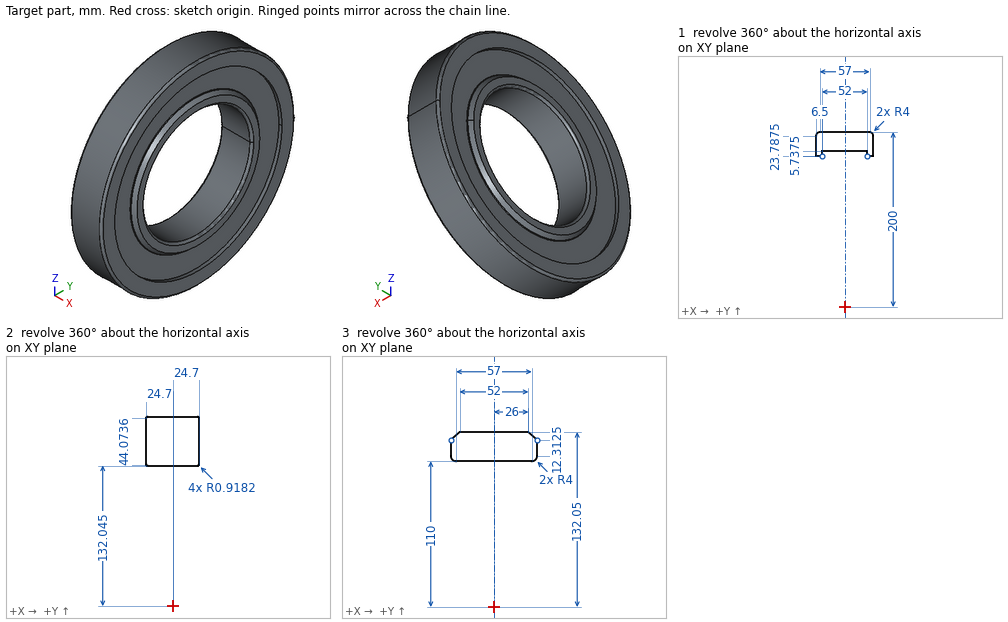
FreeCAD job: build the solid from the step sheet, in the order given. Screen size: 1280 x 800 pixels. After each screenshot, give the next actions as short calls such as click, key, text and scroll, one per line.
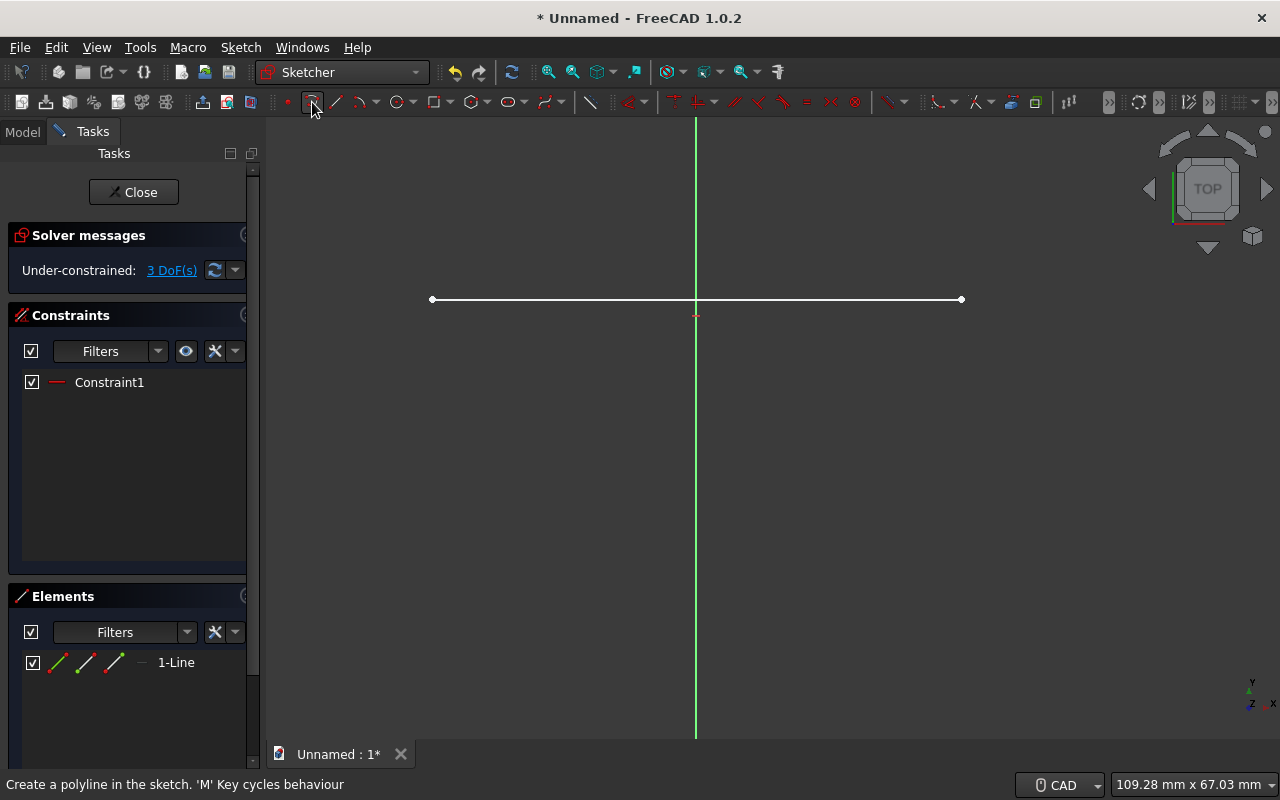
click(395, 336)
click(395, 557)
click(455, 557)
click(455, 503)
click(938, 503)
click(938, 557)
click(998, 557)
click(998, 336)
right_click(998, 336)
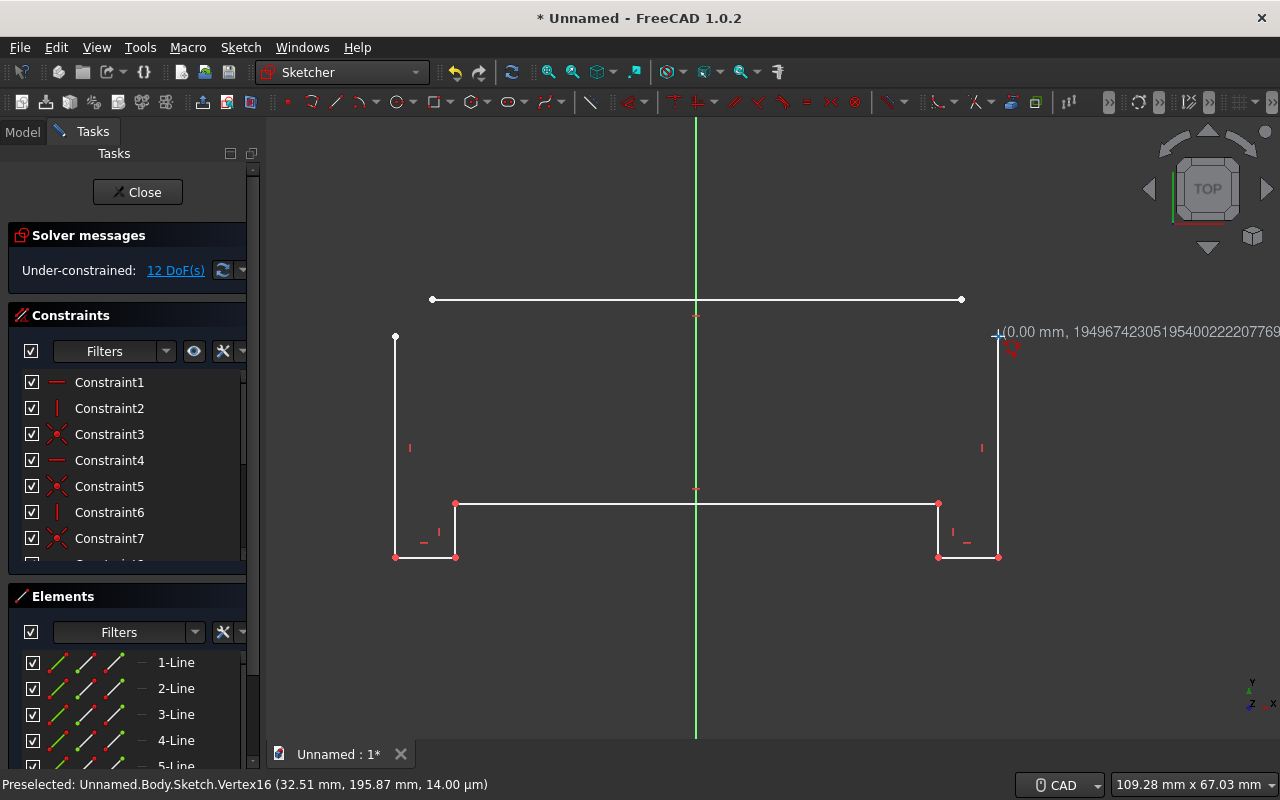
click(378, 102)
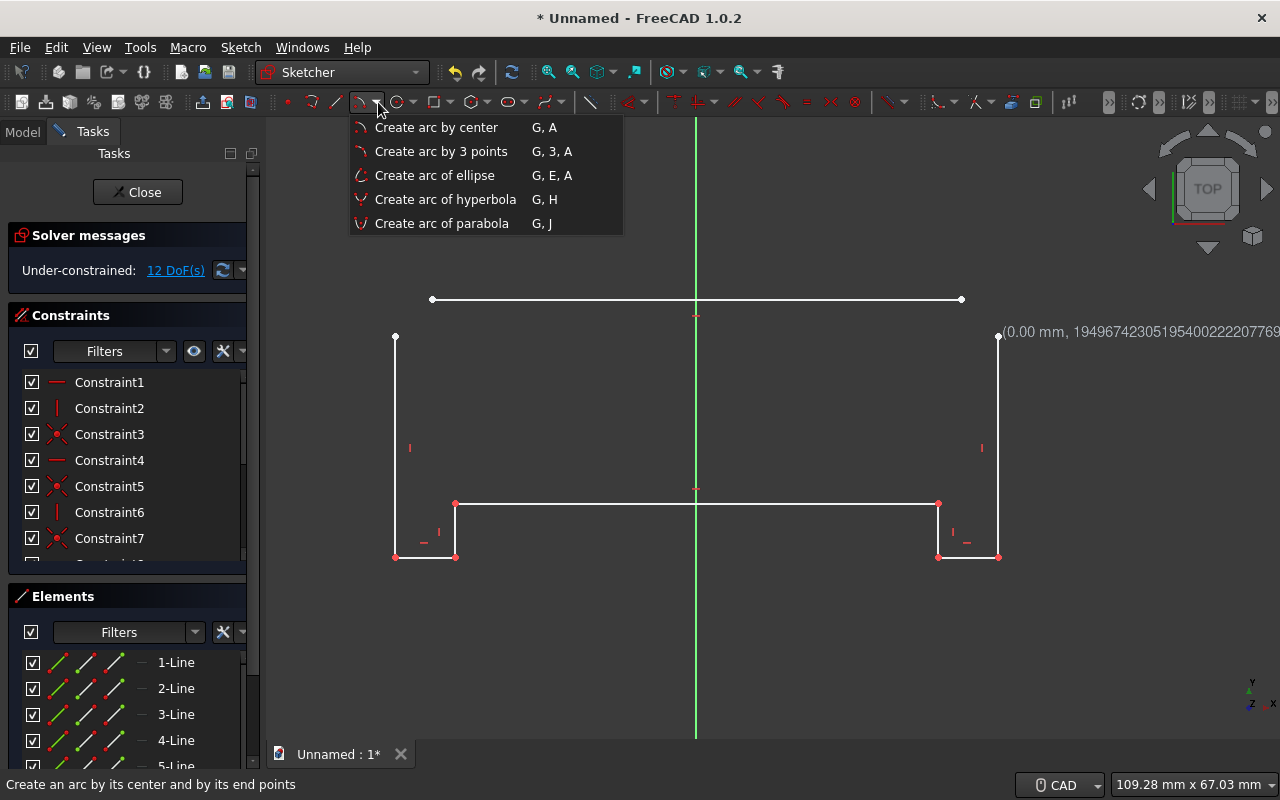
click(486, 151)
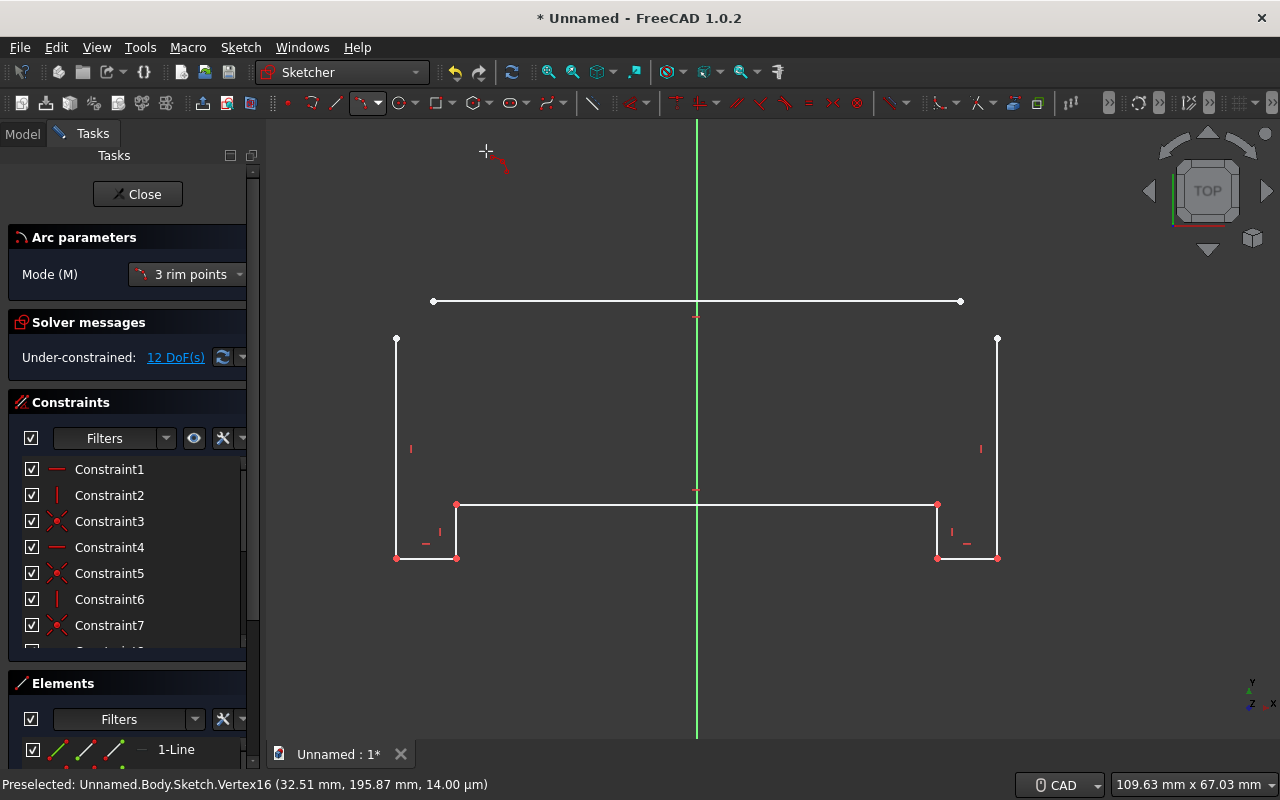
click(433, 301)
click(396, 338)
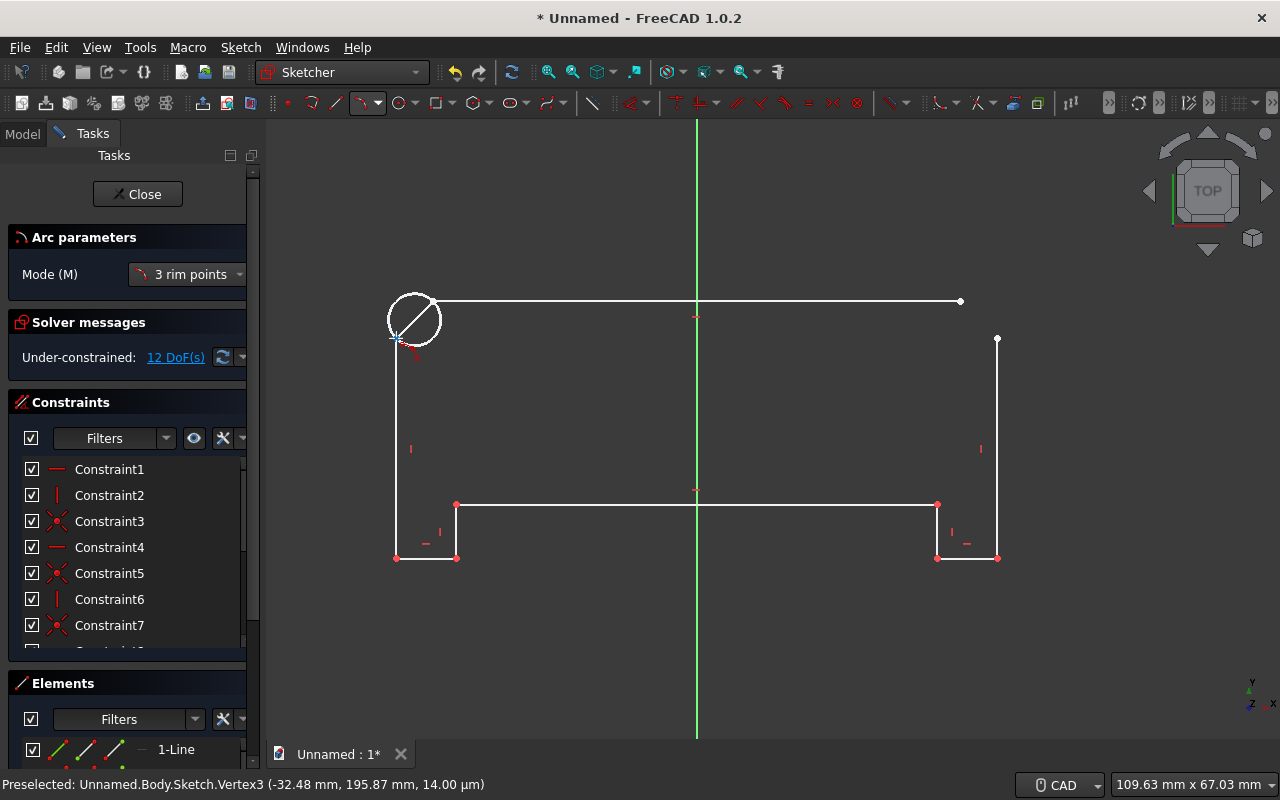
scroll(407, 311, up, 2)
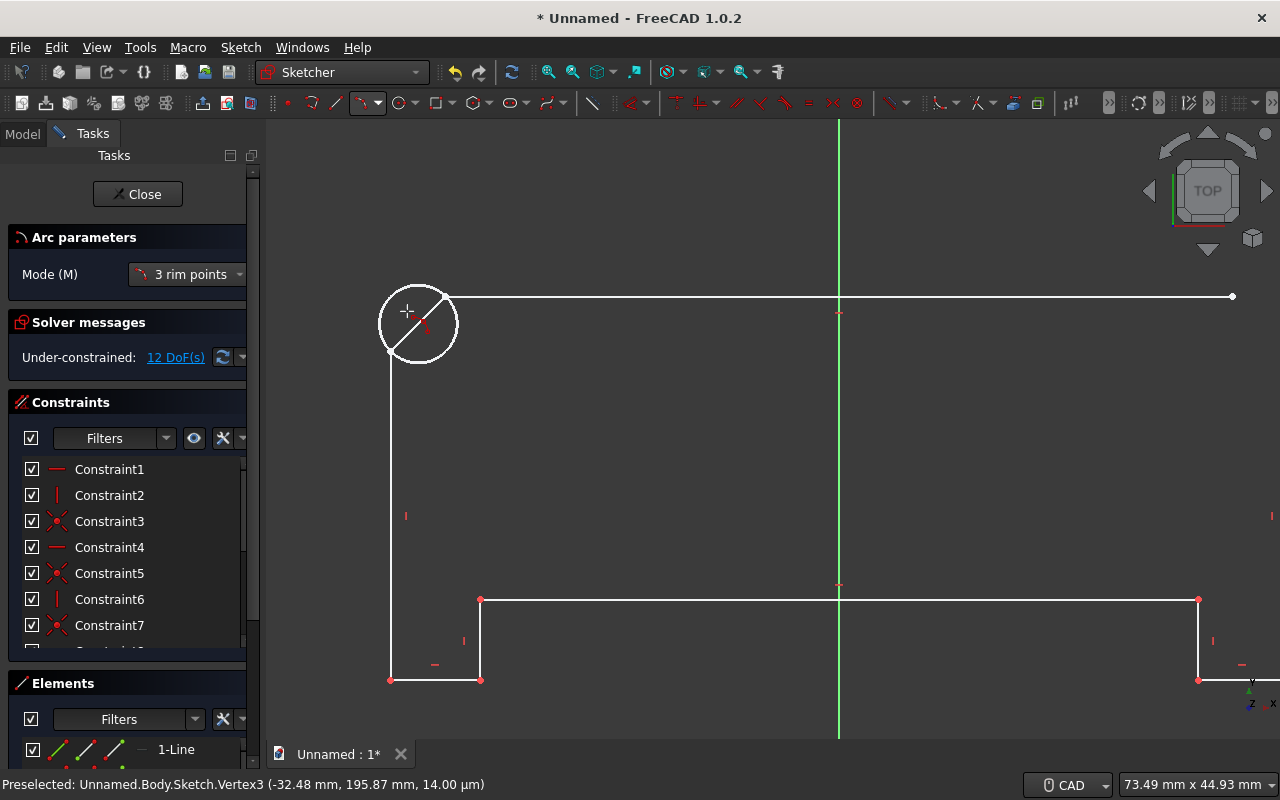
click(407, 311)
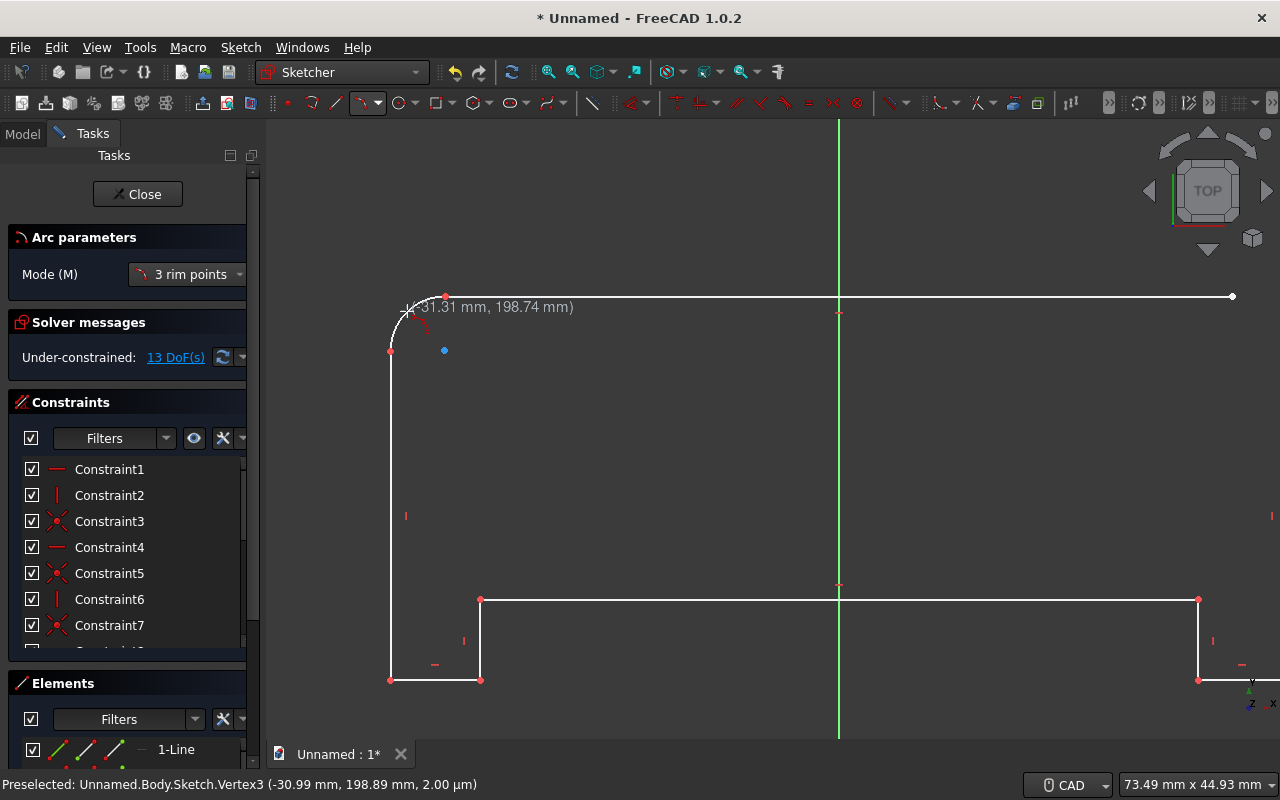
scroll(431, 312, down, 2)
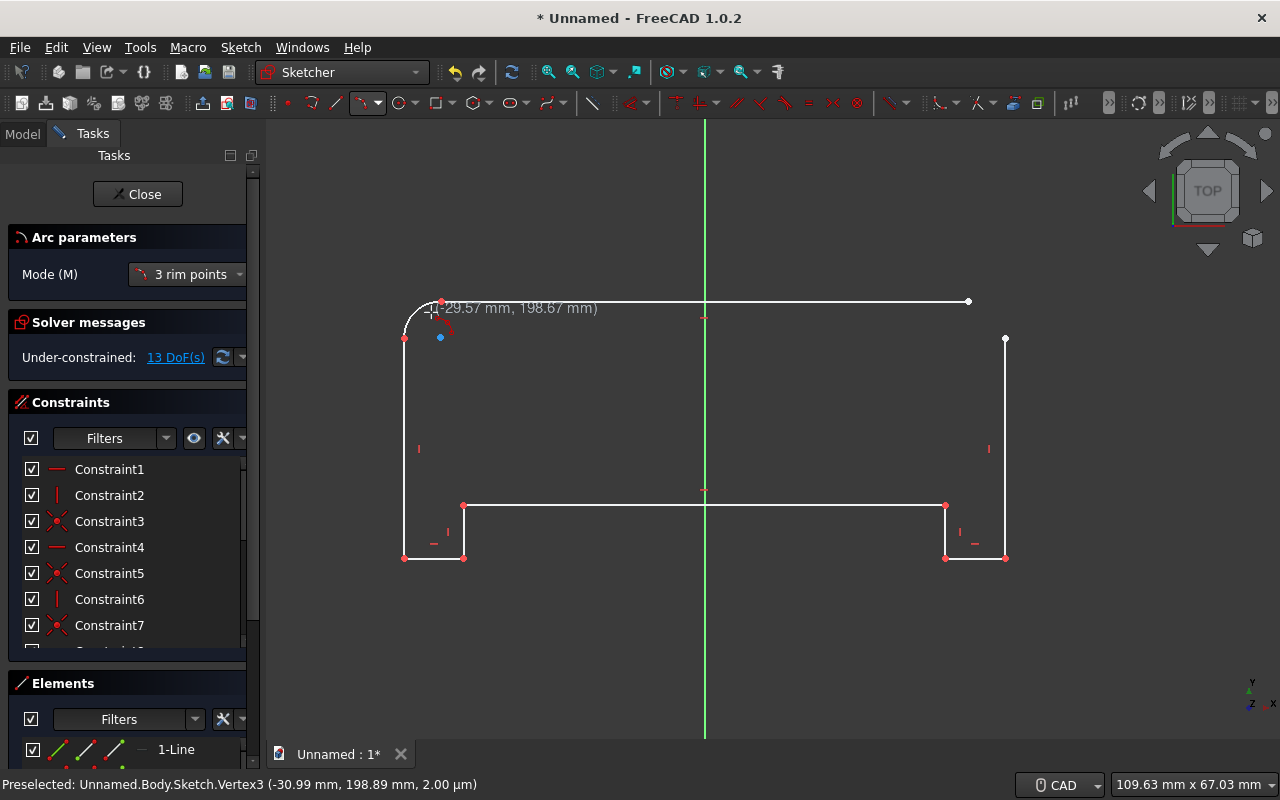
click(1005, 339)
click(968, 302)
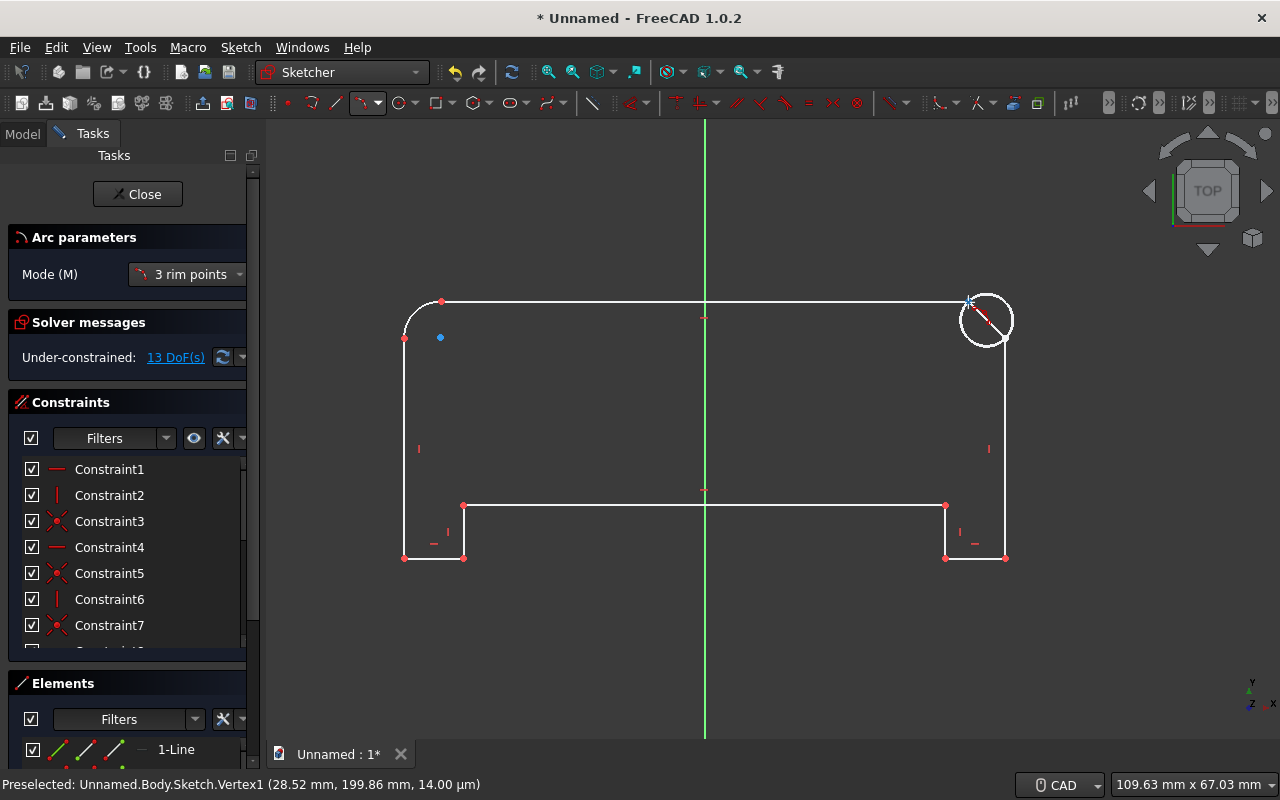
scroll(994, 311, up, 2)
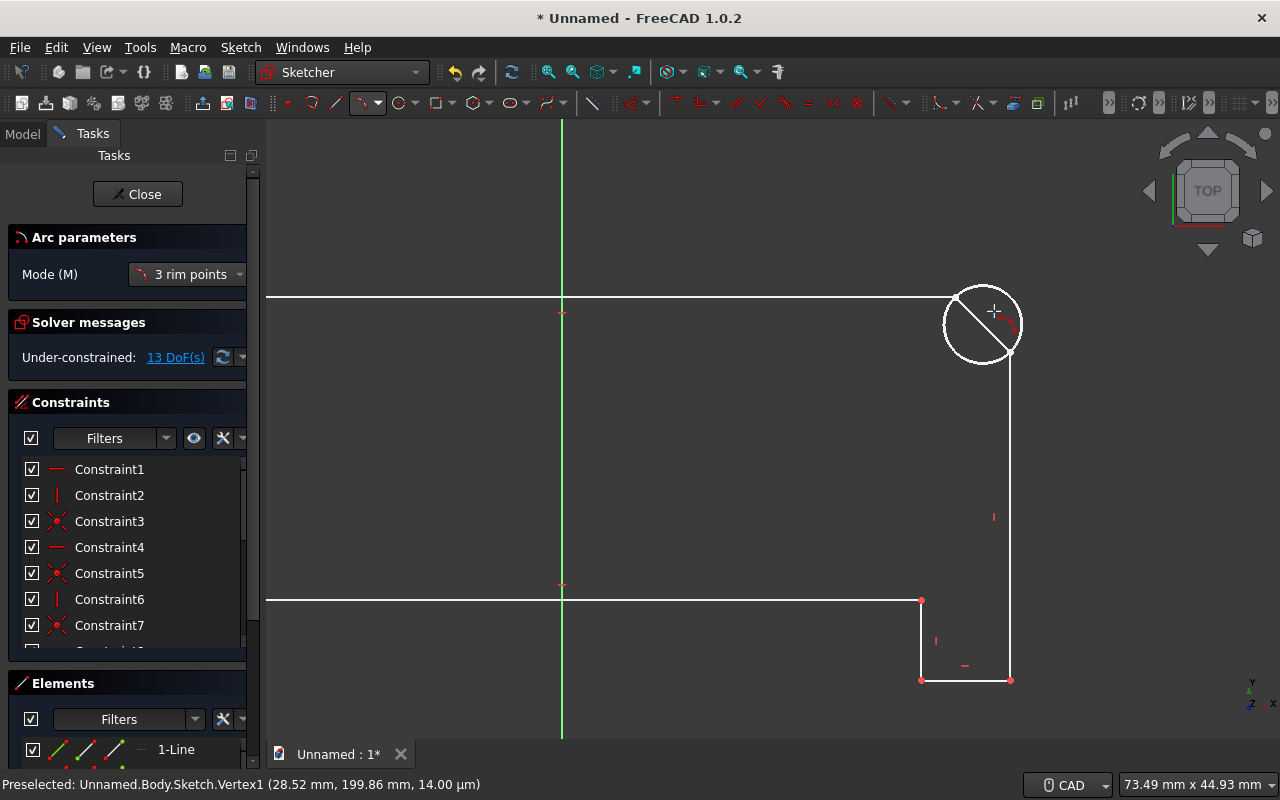
click(994, 311)
key(Escape)